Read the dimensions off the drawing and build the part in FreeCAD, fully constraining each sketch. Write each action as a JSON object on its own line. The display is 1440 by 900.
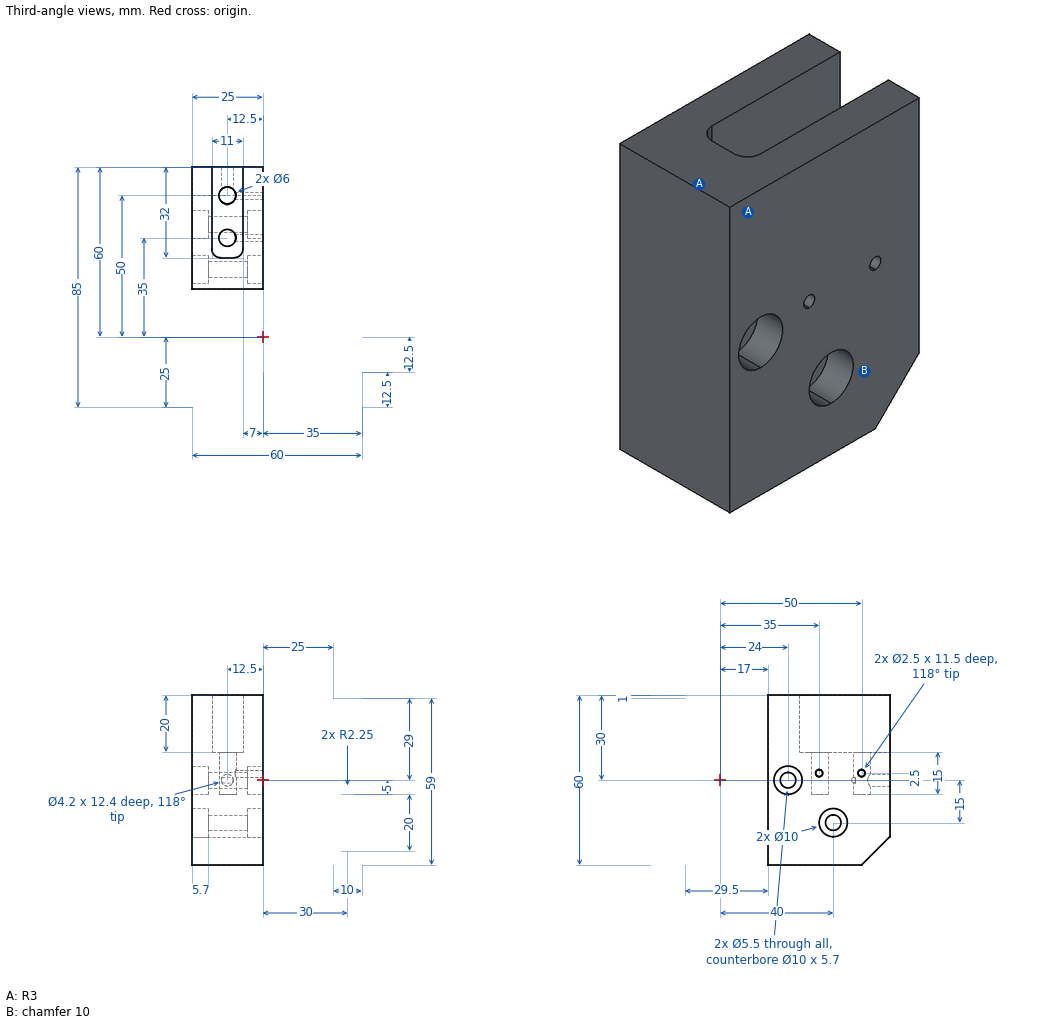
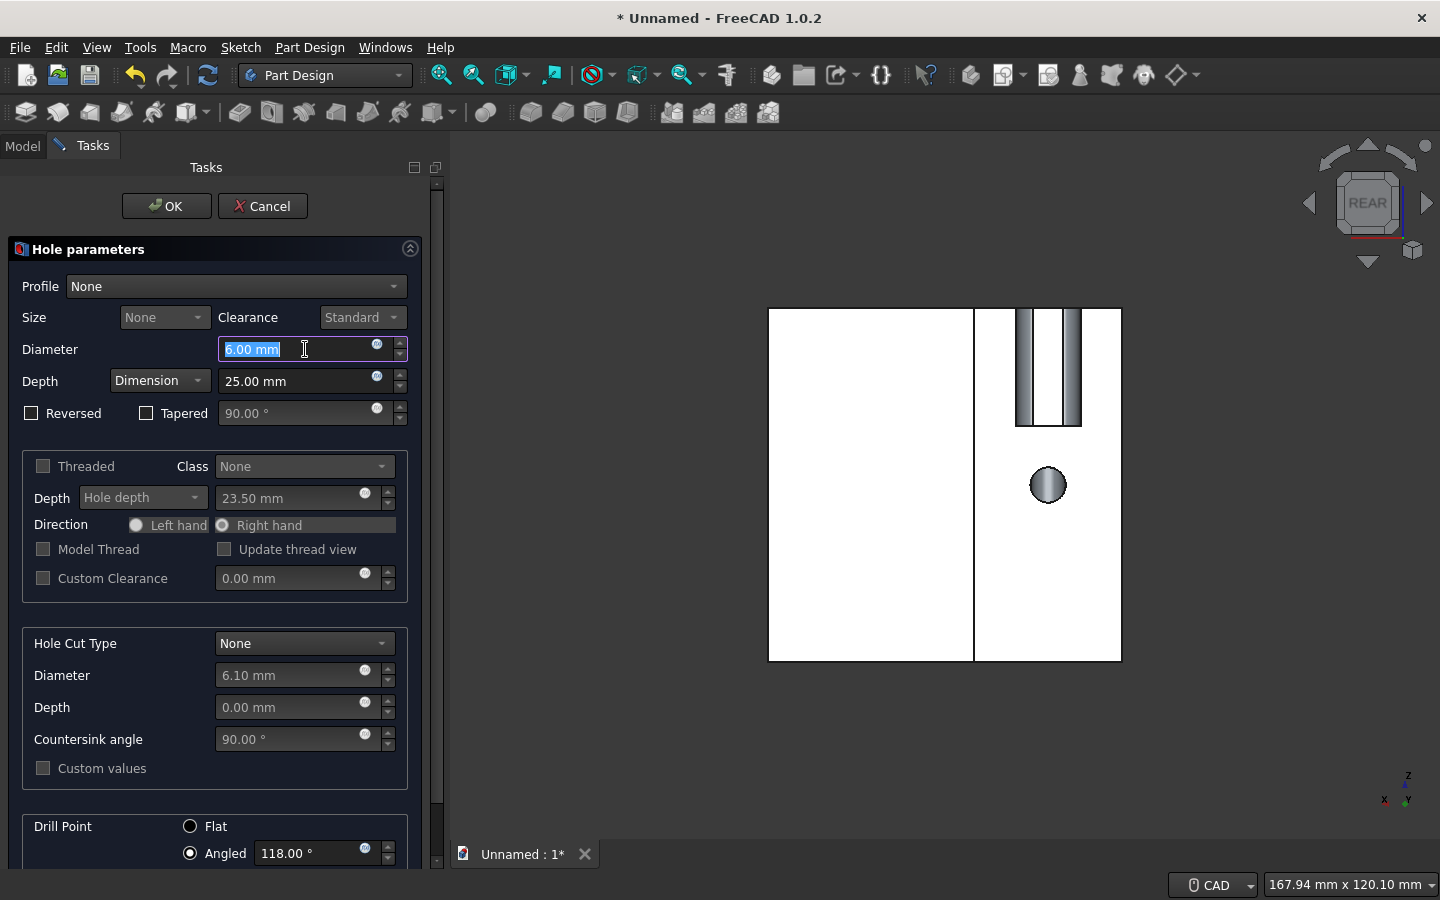
{"action": "type", "text": "4.2"}
{"action": "key", "text": "Tab"}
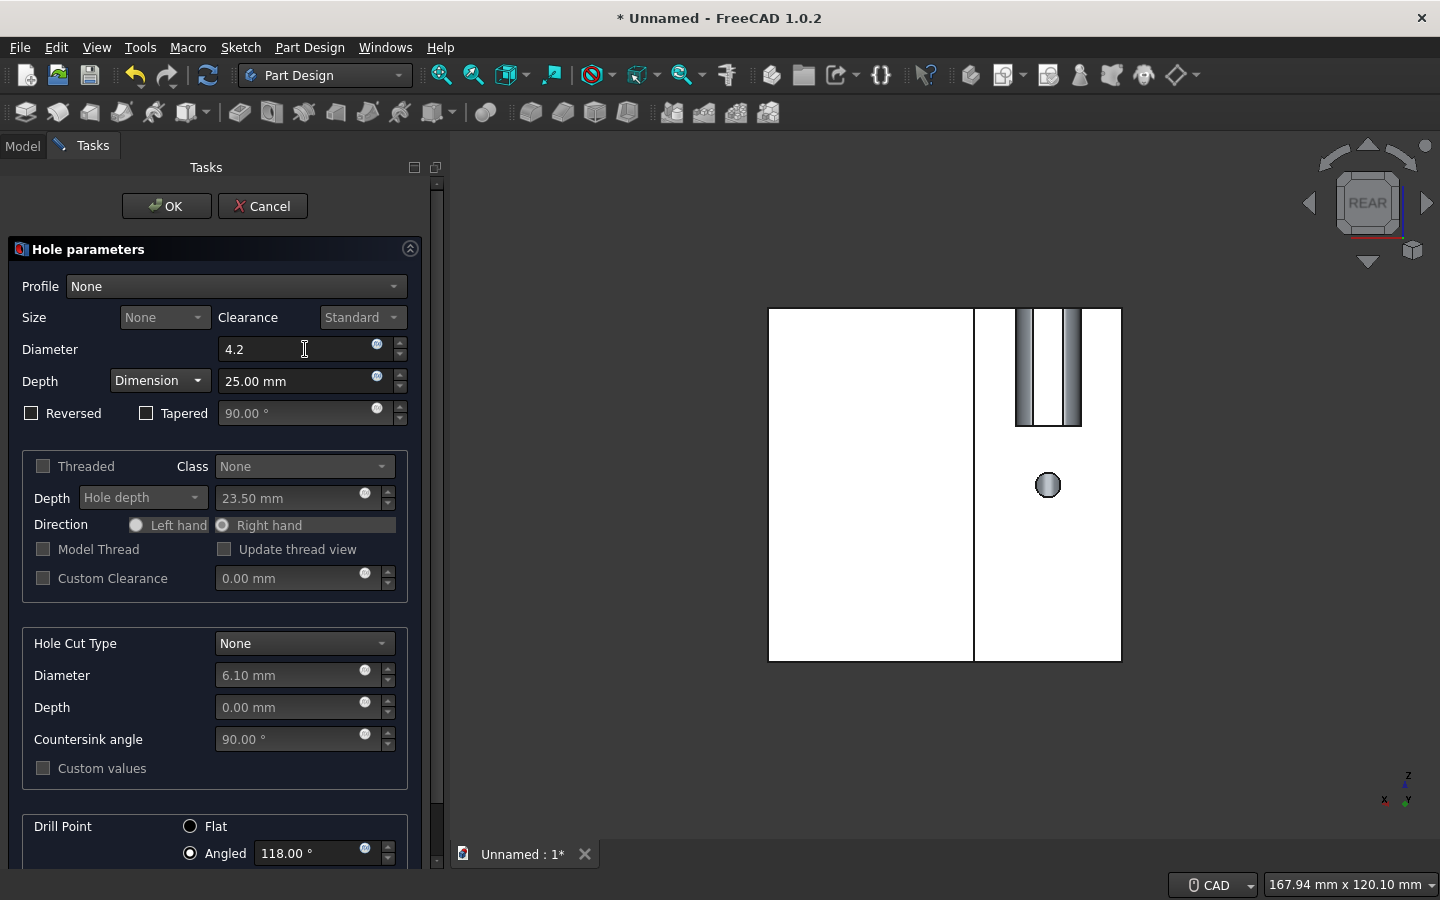
{"action": "triple_click", "coordinate": [305, 381]}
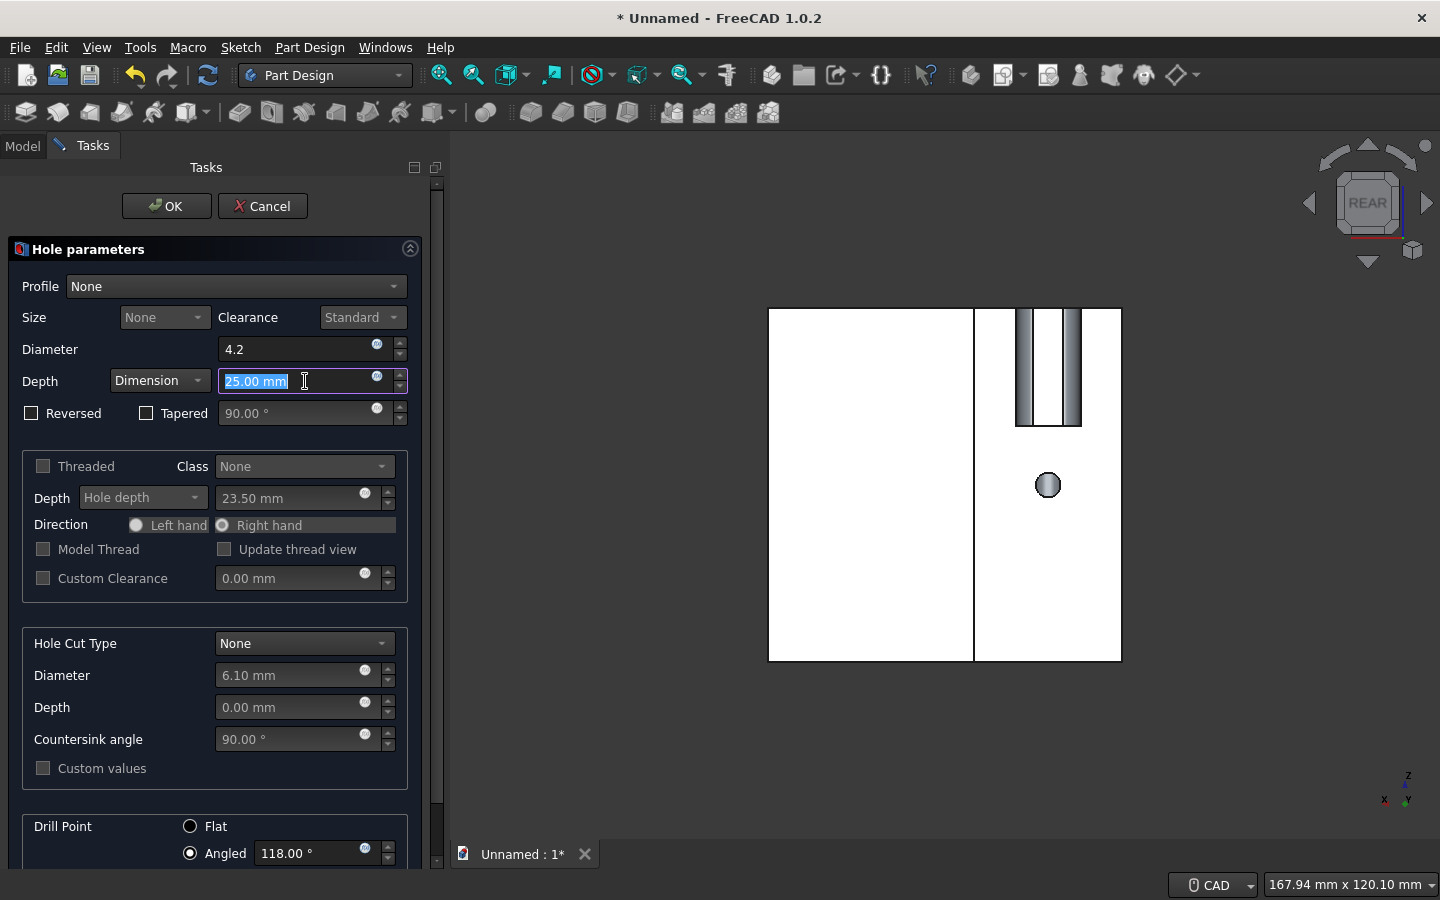
{"action": "type", "text": "12.4"}
{"action": "key", "text": "Tab"}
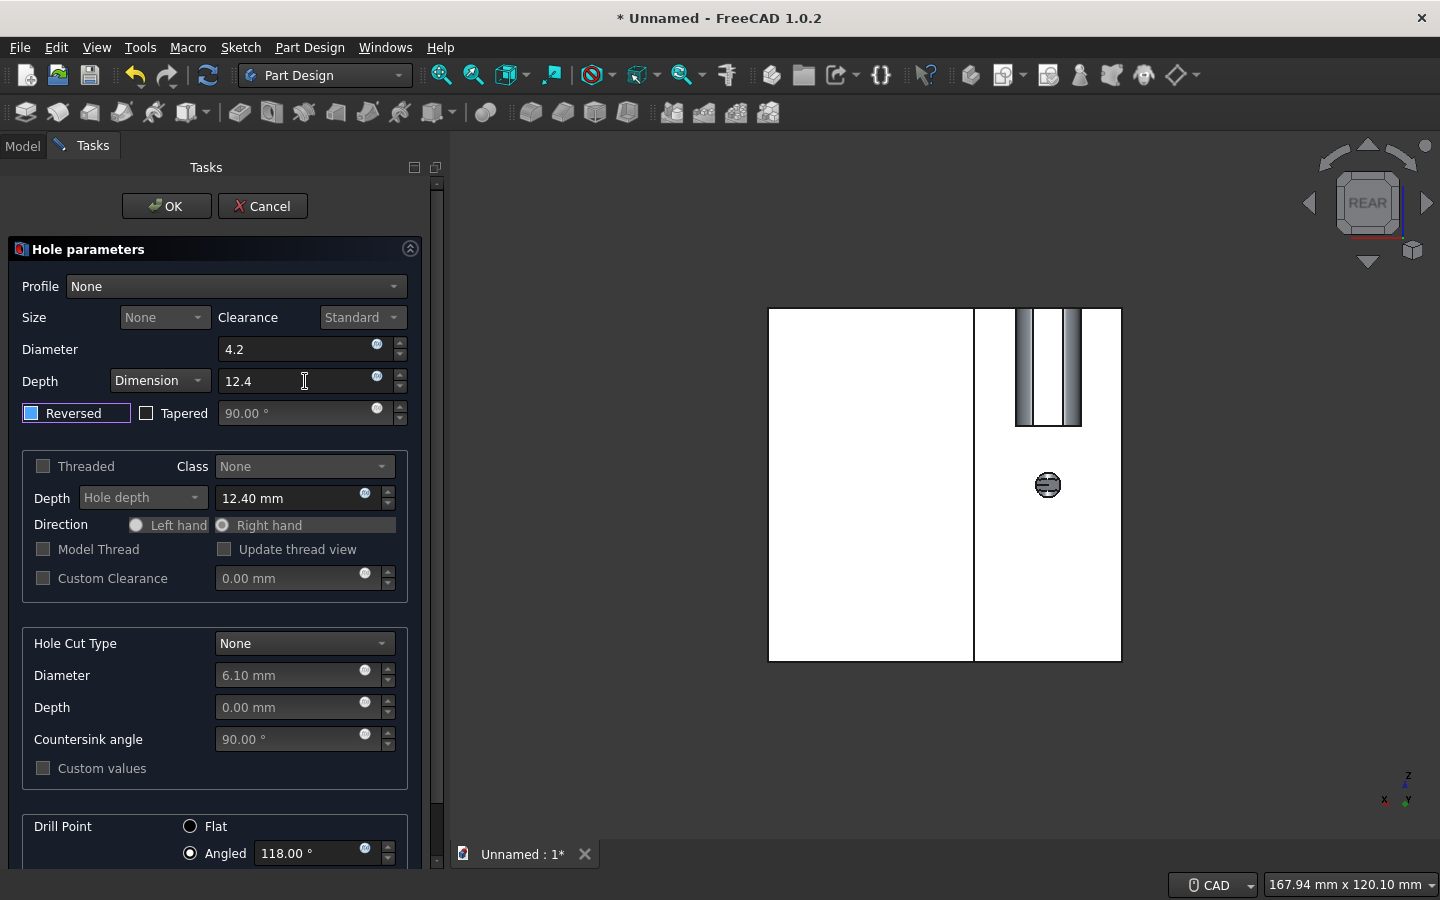
{"action": "left_click", "coordinate": [167, 206]}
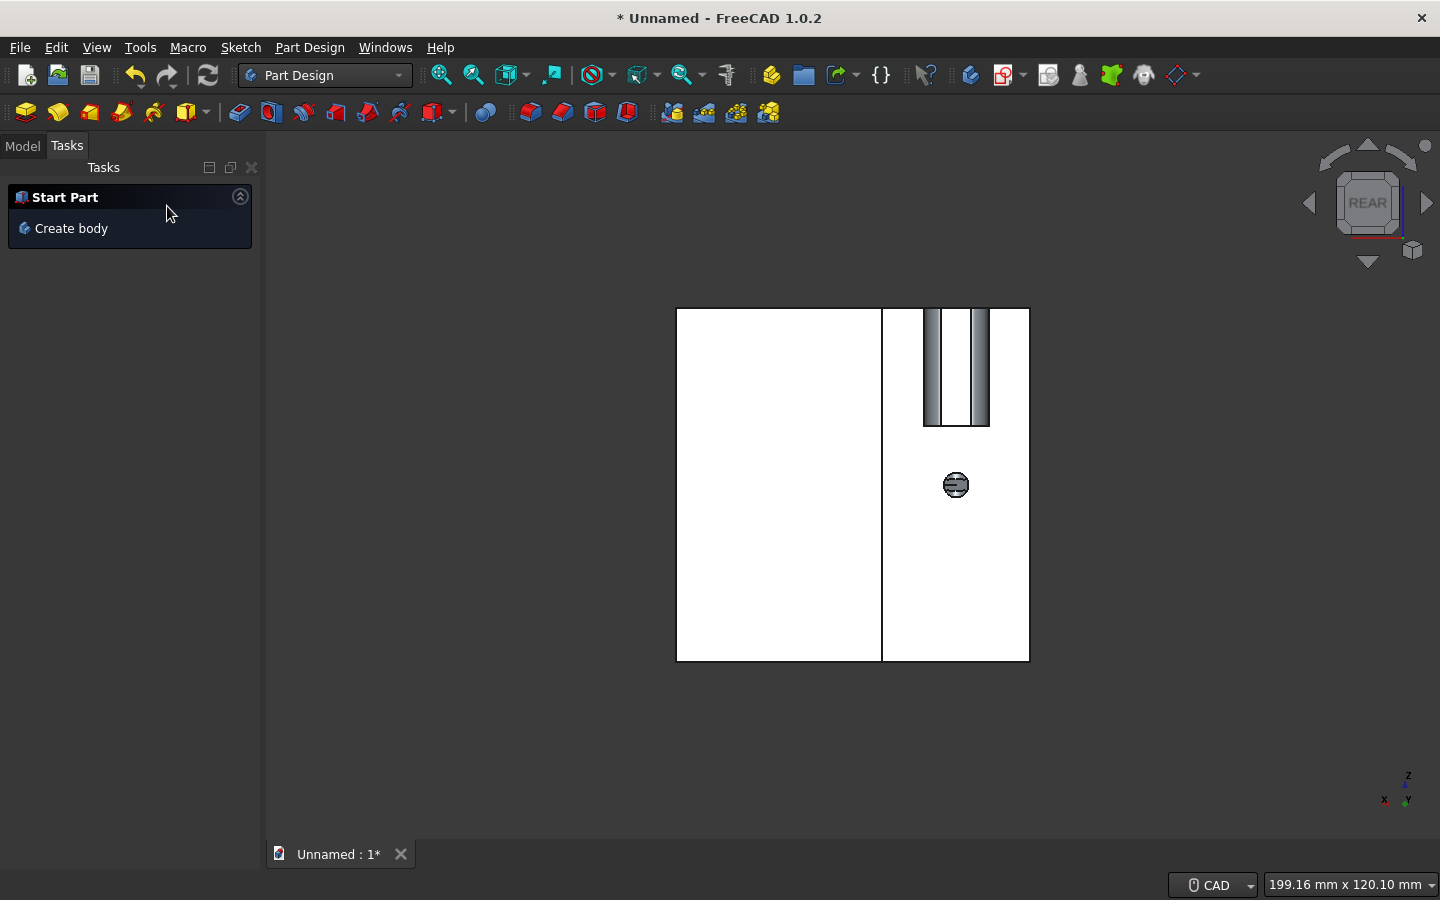
{"action": "key", "text": "0"}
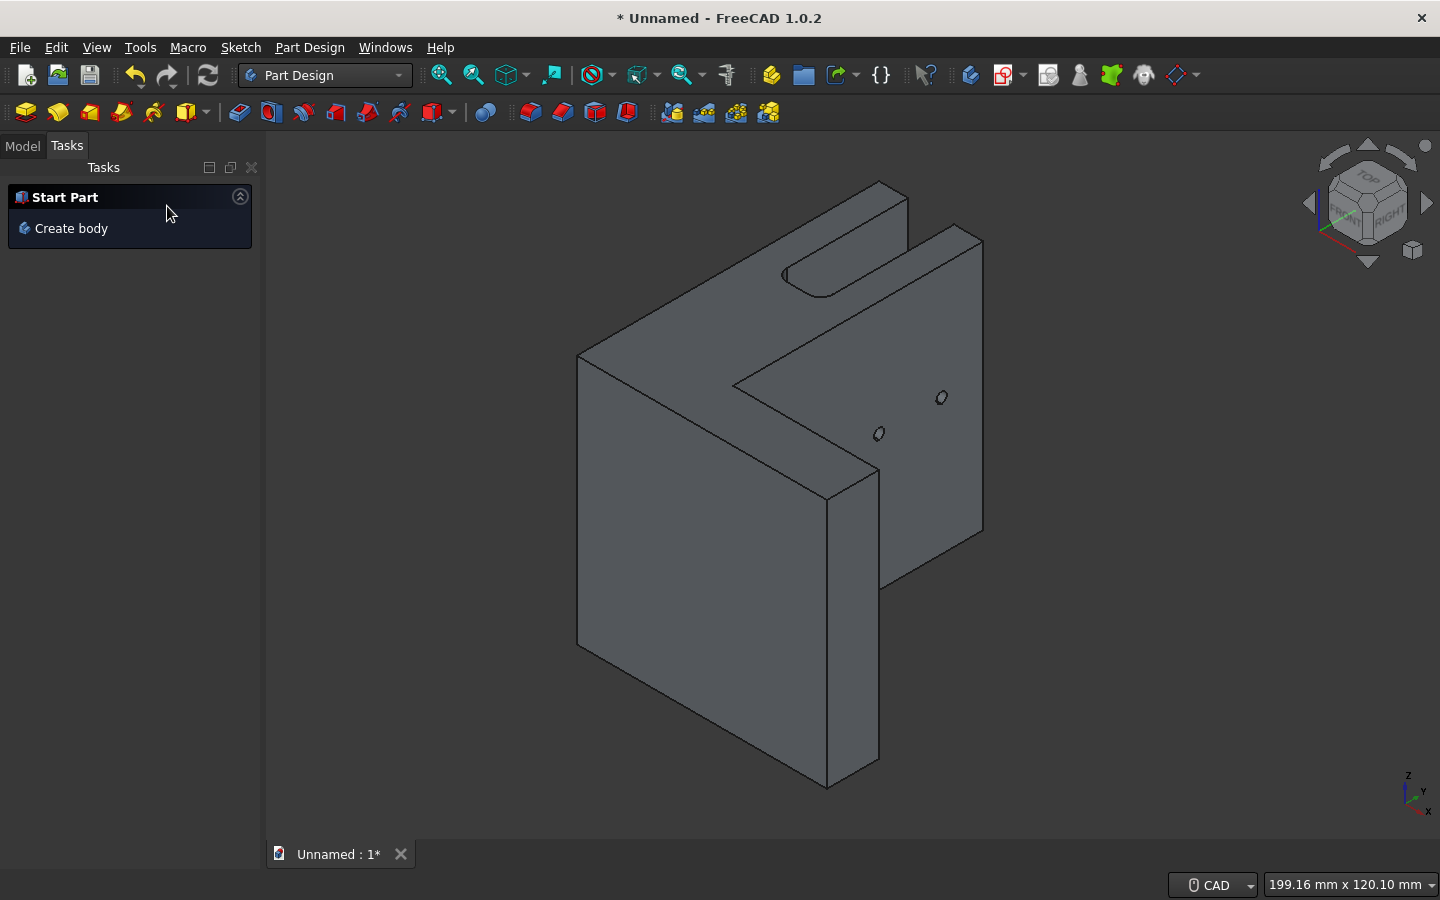
{"action": "left_click", "coordinate": [702, 571]}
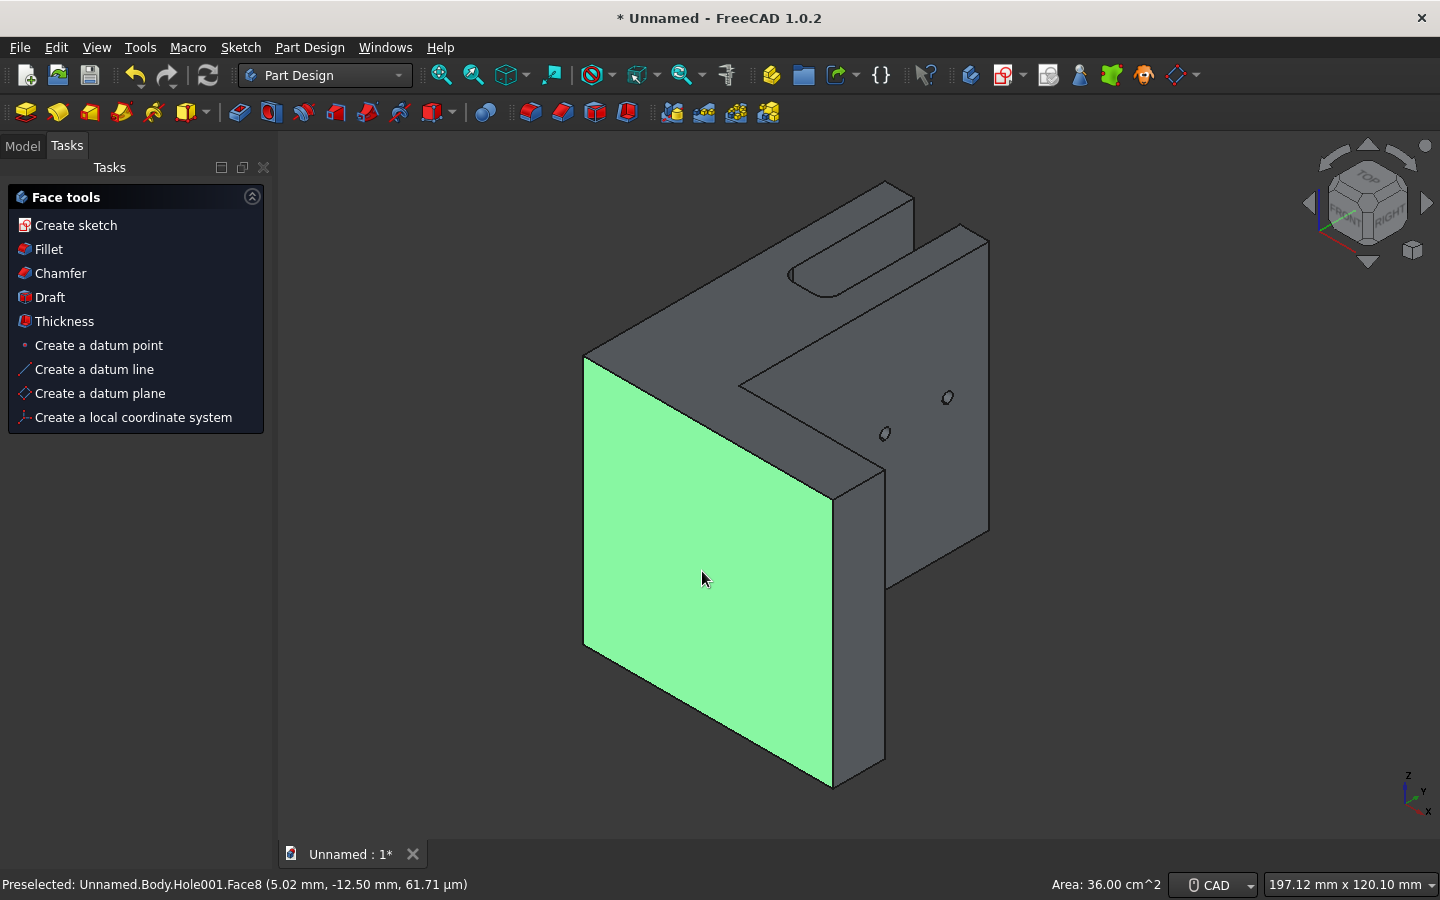
{"action": "left_click", "coordinate": [1004, 76]}